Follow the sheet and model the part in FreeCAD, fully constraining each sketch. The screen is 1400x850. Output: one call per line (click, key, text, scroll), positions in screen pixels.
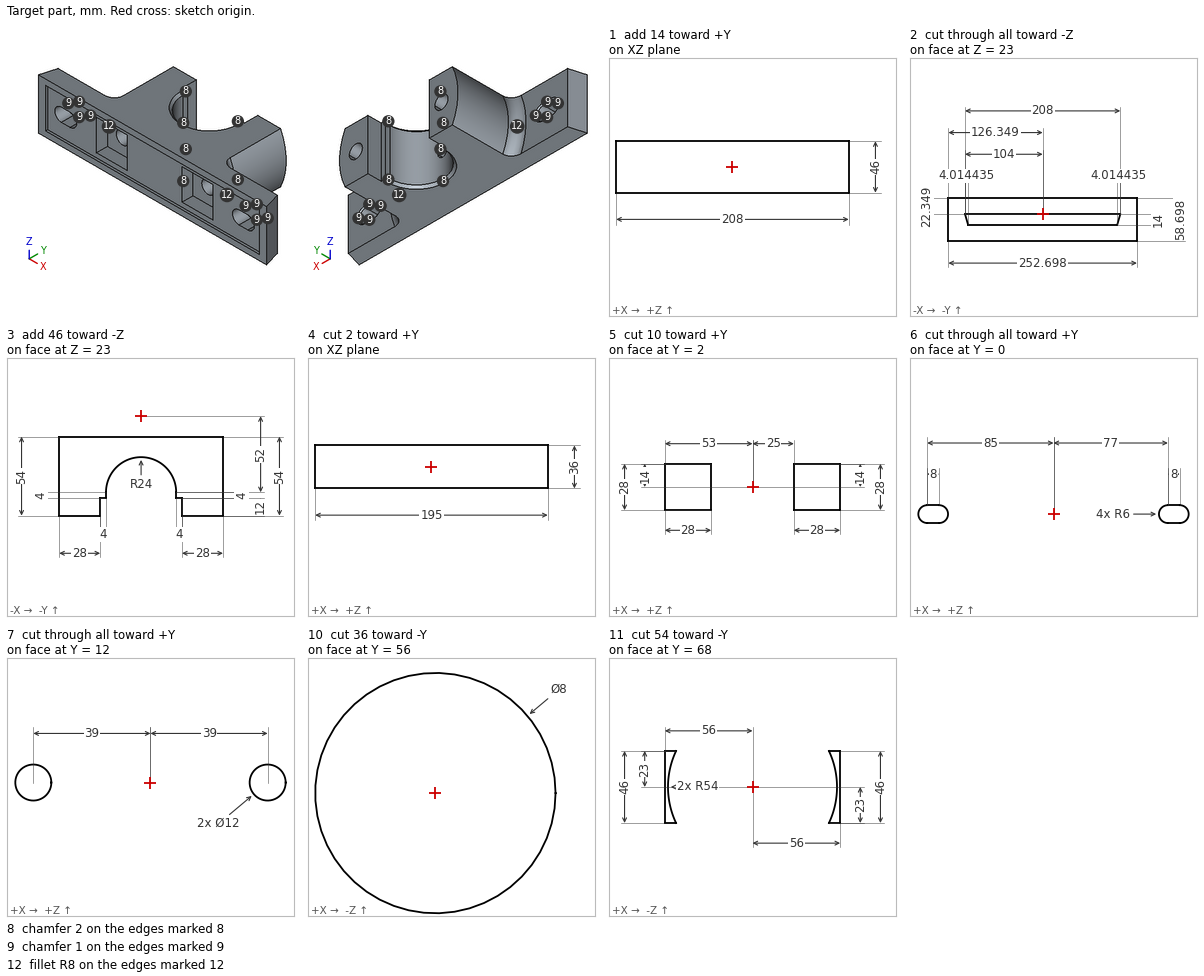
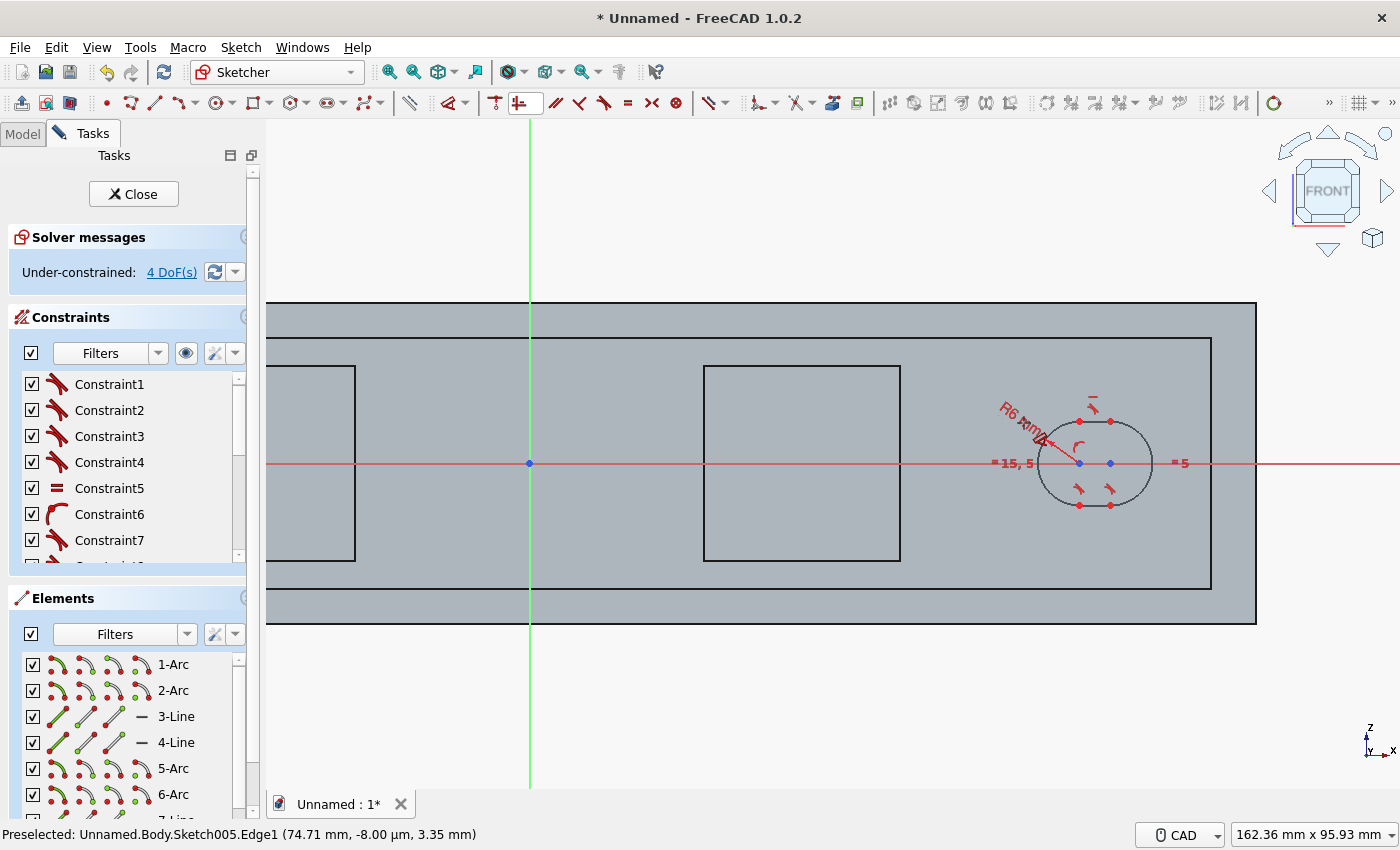
scroll(1089, 422, up, 3)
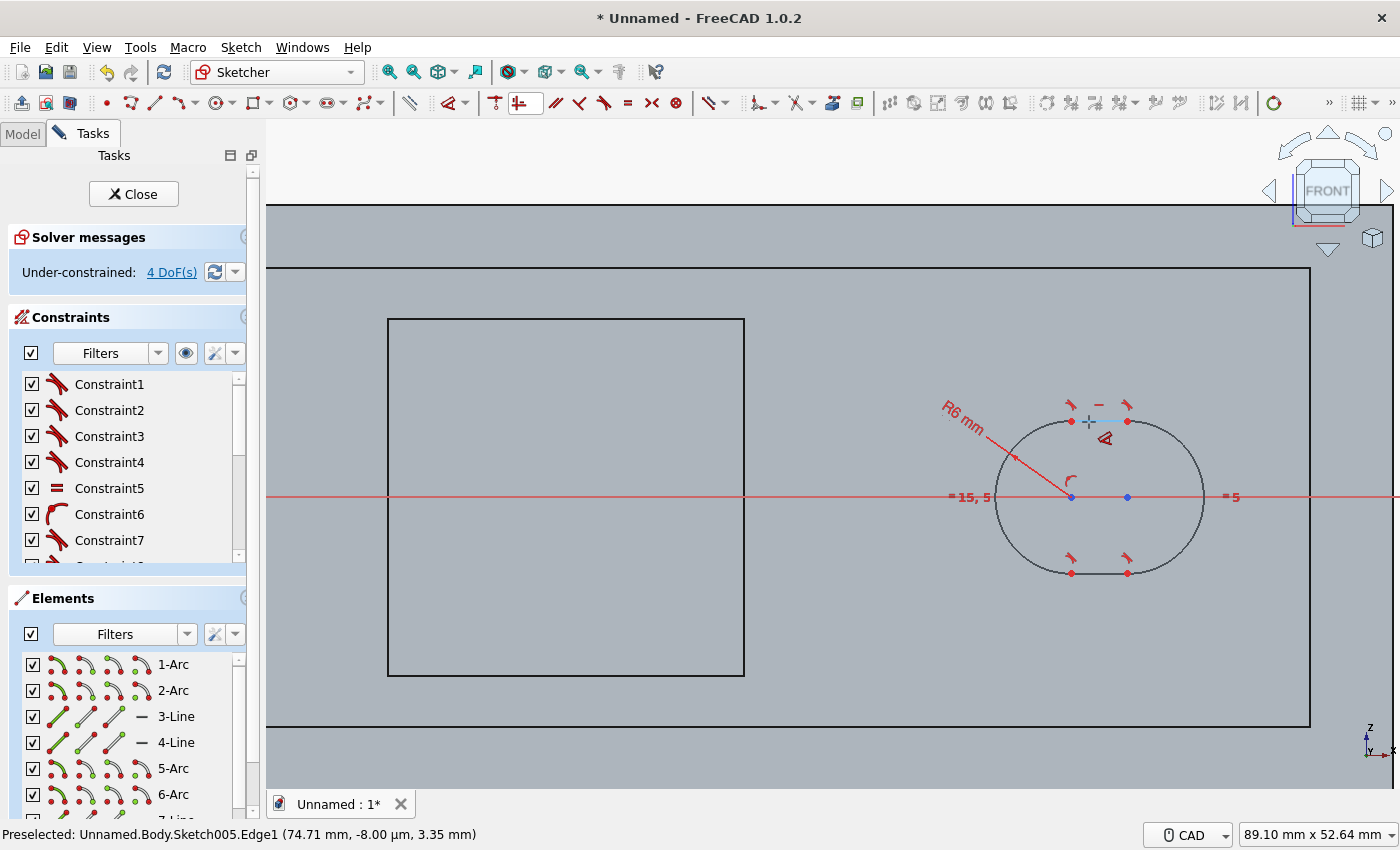
click(1088, 421)
click(1100, 387)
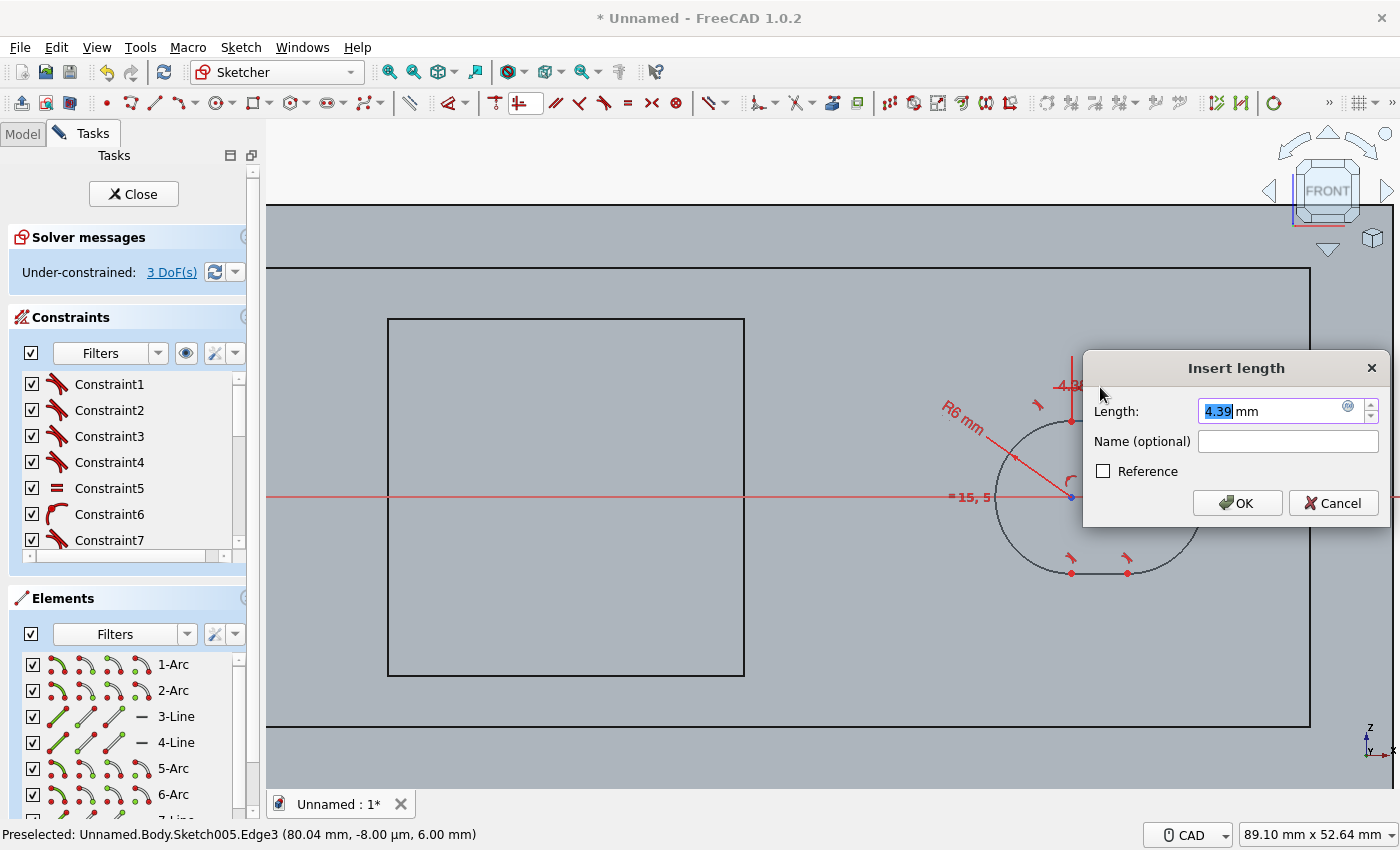
text(8)
key(Return)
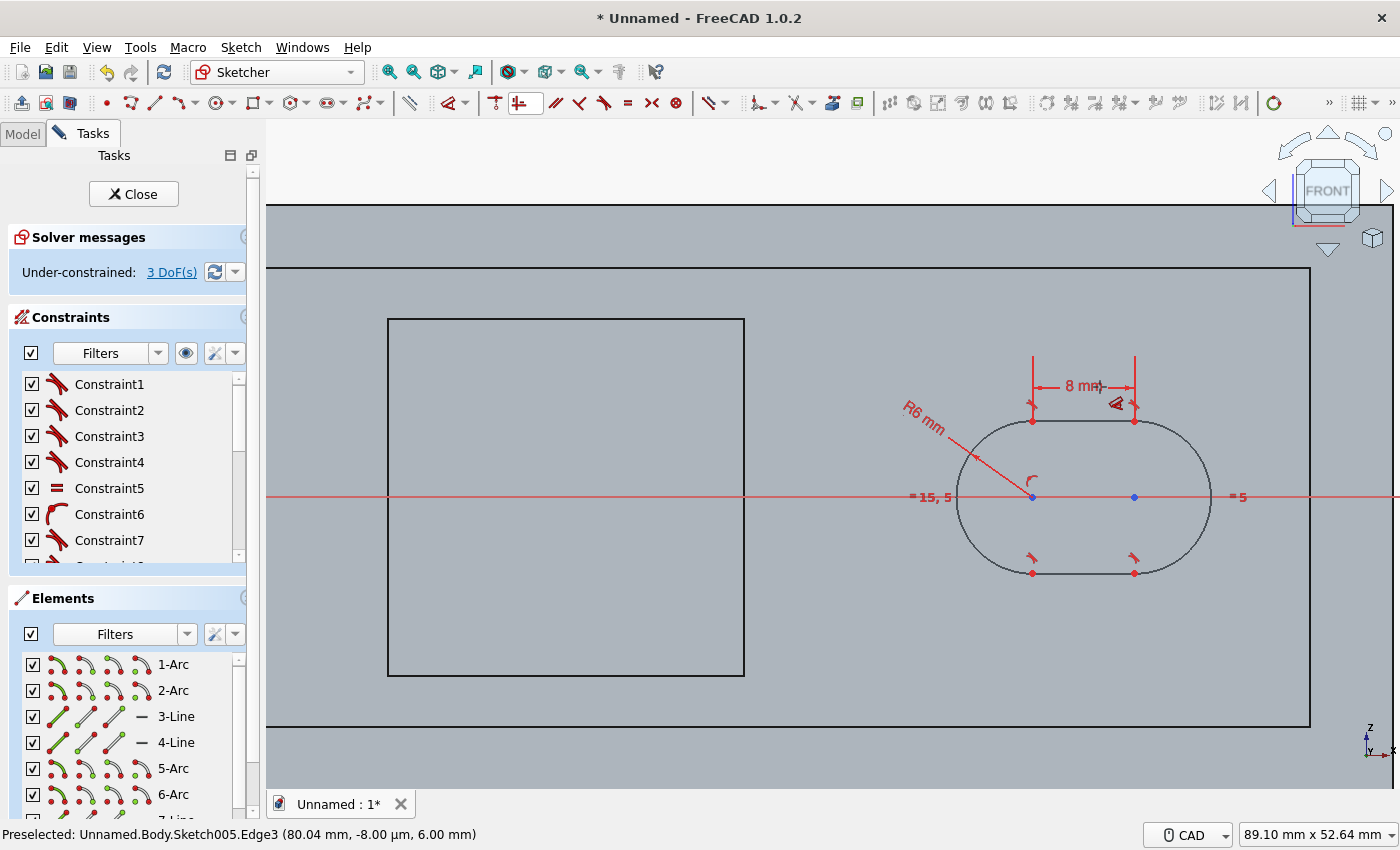
scroll(1064, 435, down, 6)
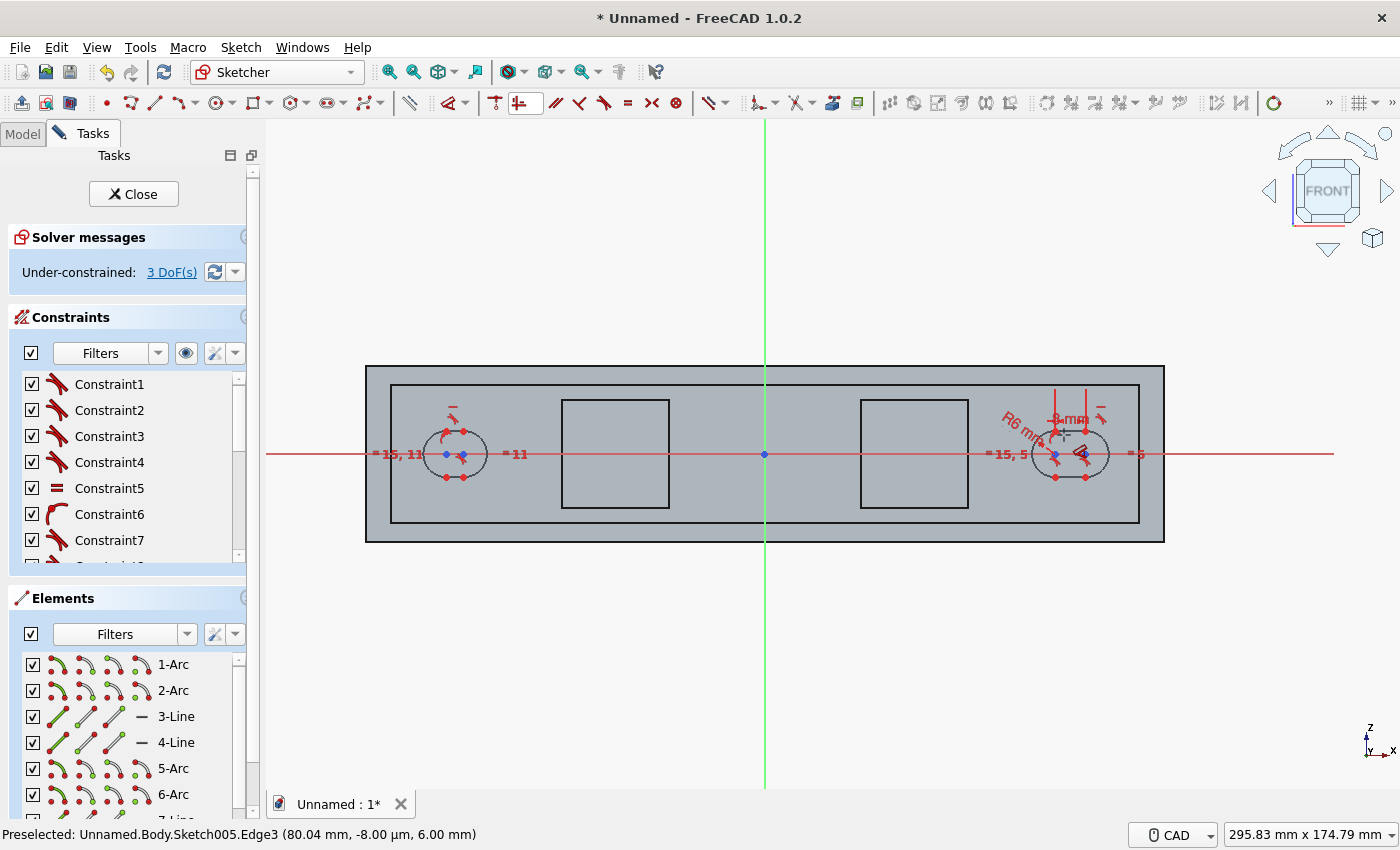
scroll(452, 431, up, 5)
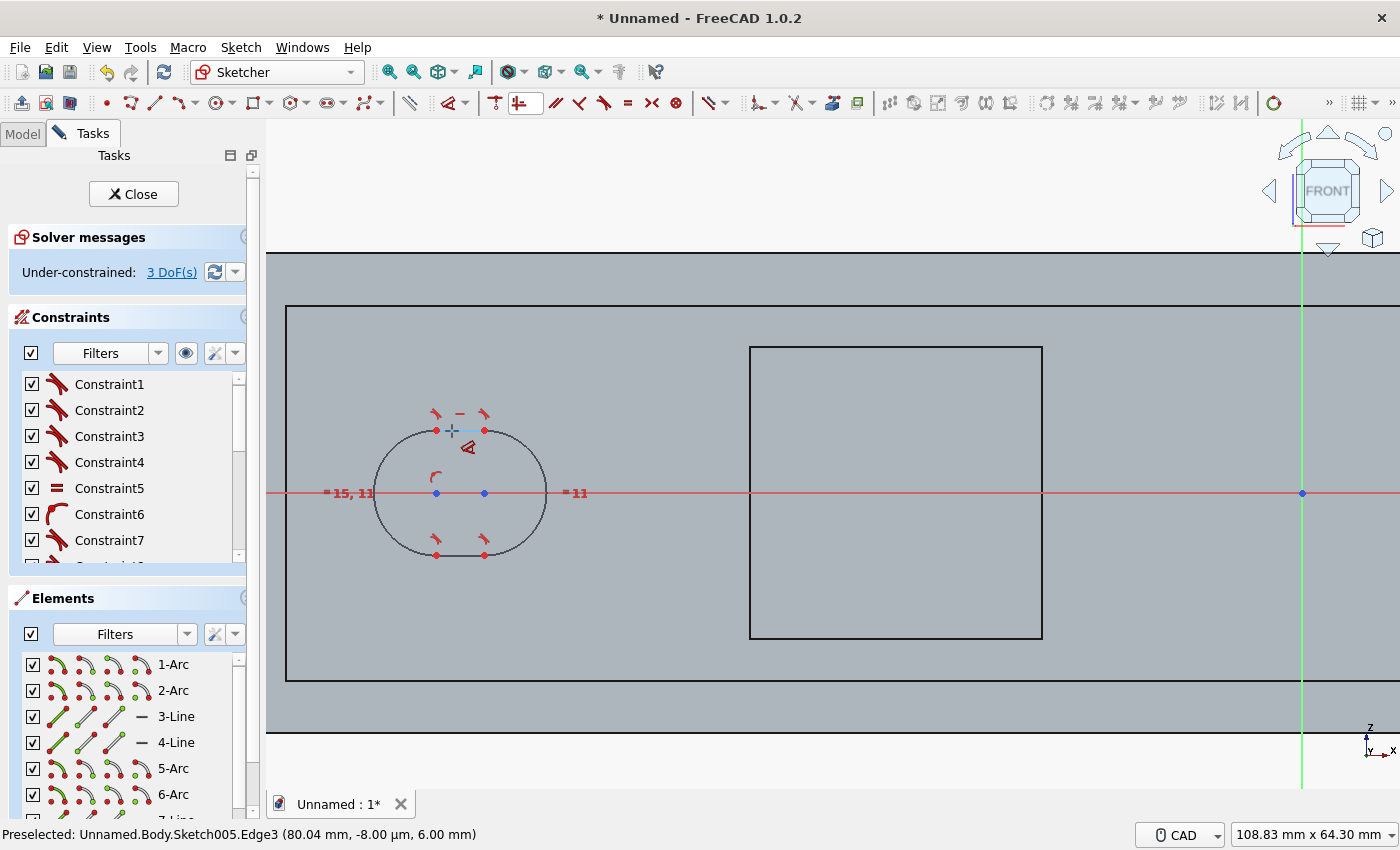
click(451, 431)
click(460, 397)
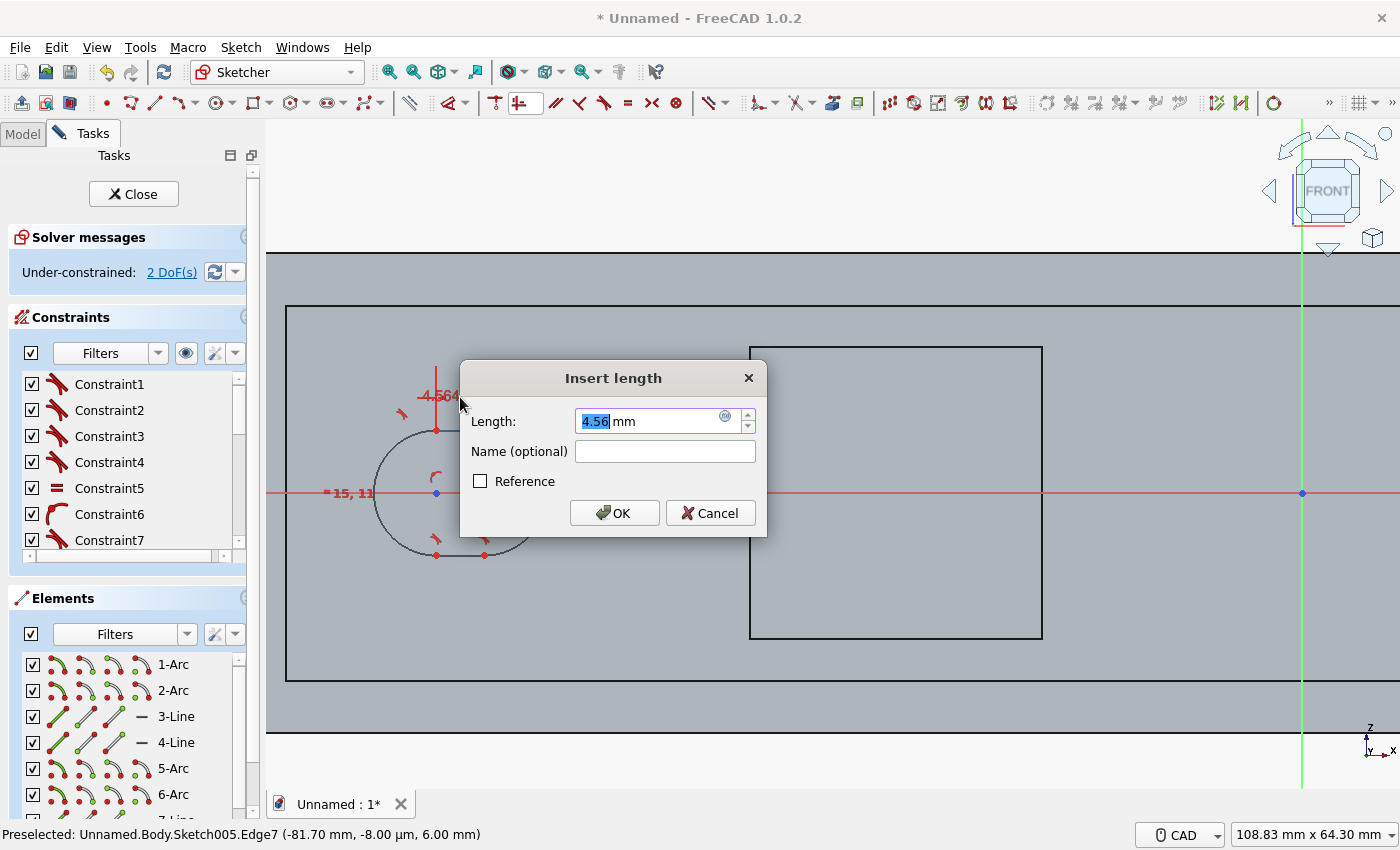
text(8)
key(Return)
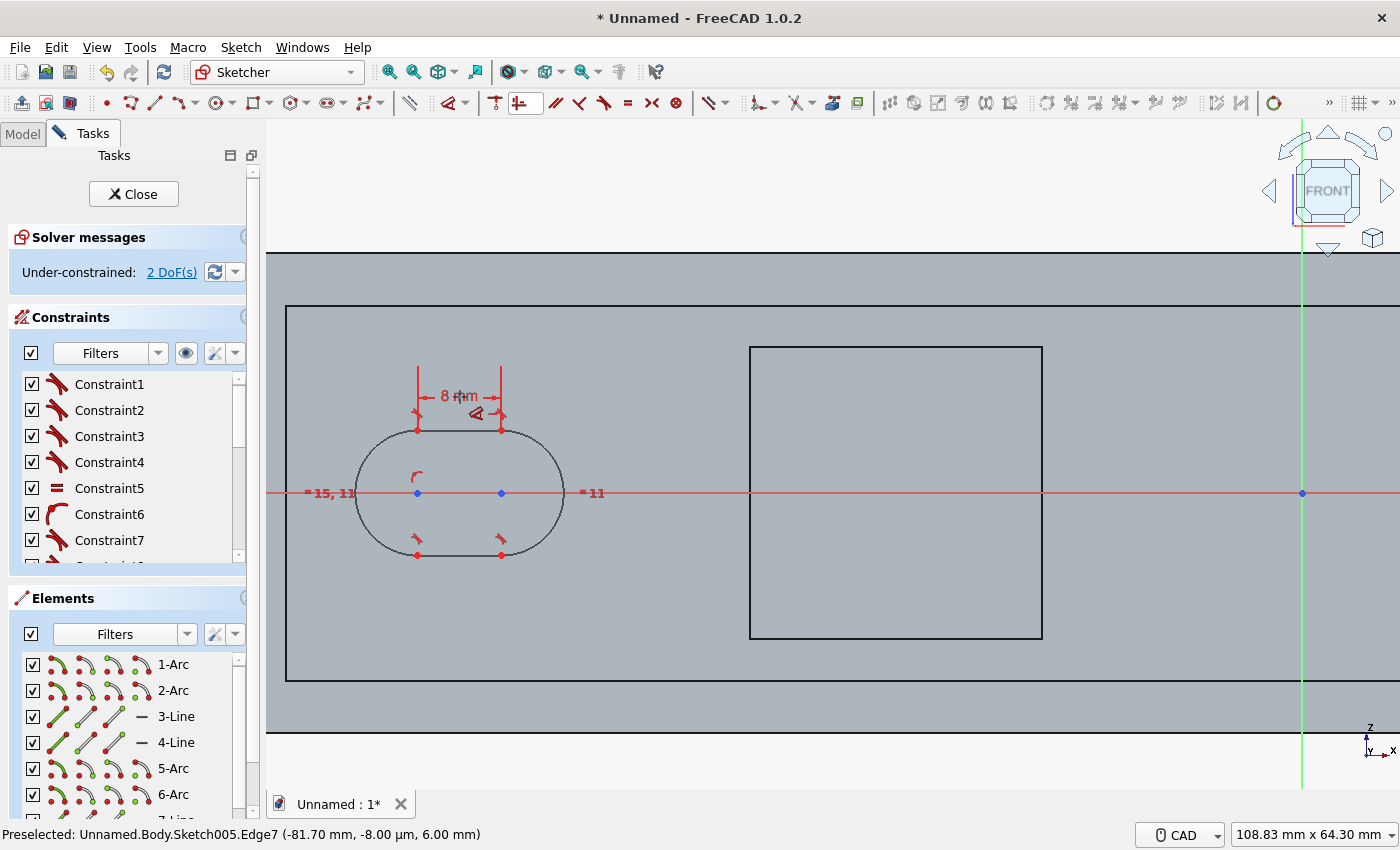
scroll(451, 431, down, 5)